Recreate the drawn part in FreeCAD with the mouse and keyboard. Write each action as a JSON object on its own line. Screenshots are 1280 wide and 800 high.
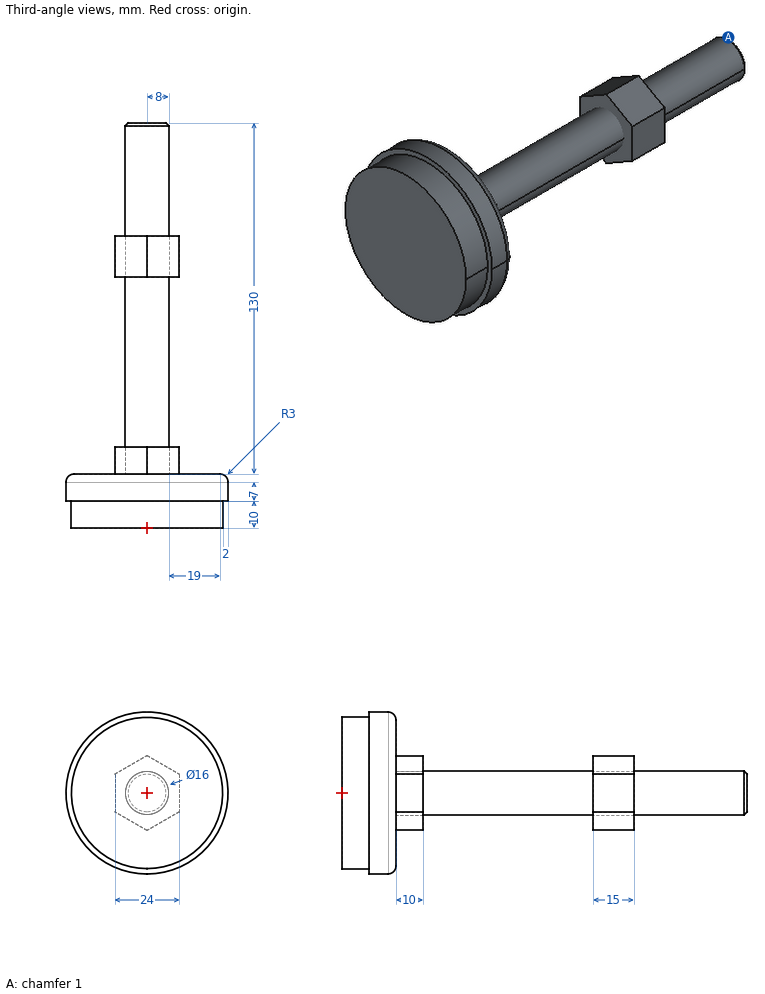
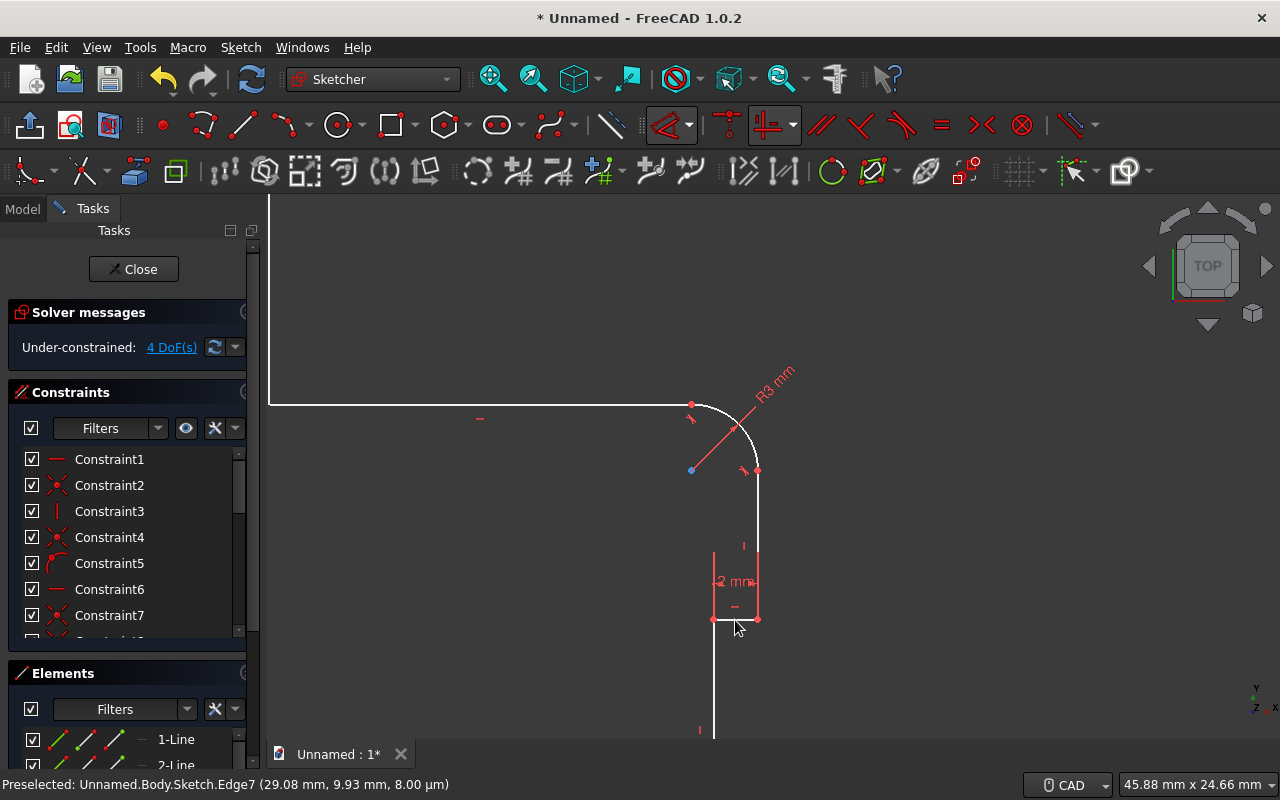
{"action": "scroll", "coordinate": [739, 627], "scroll_direction": "down", "scroll_amount": 11}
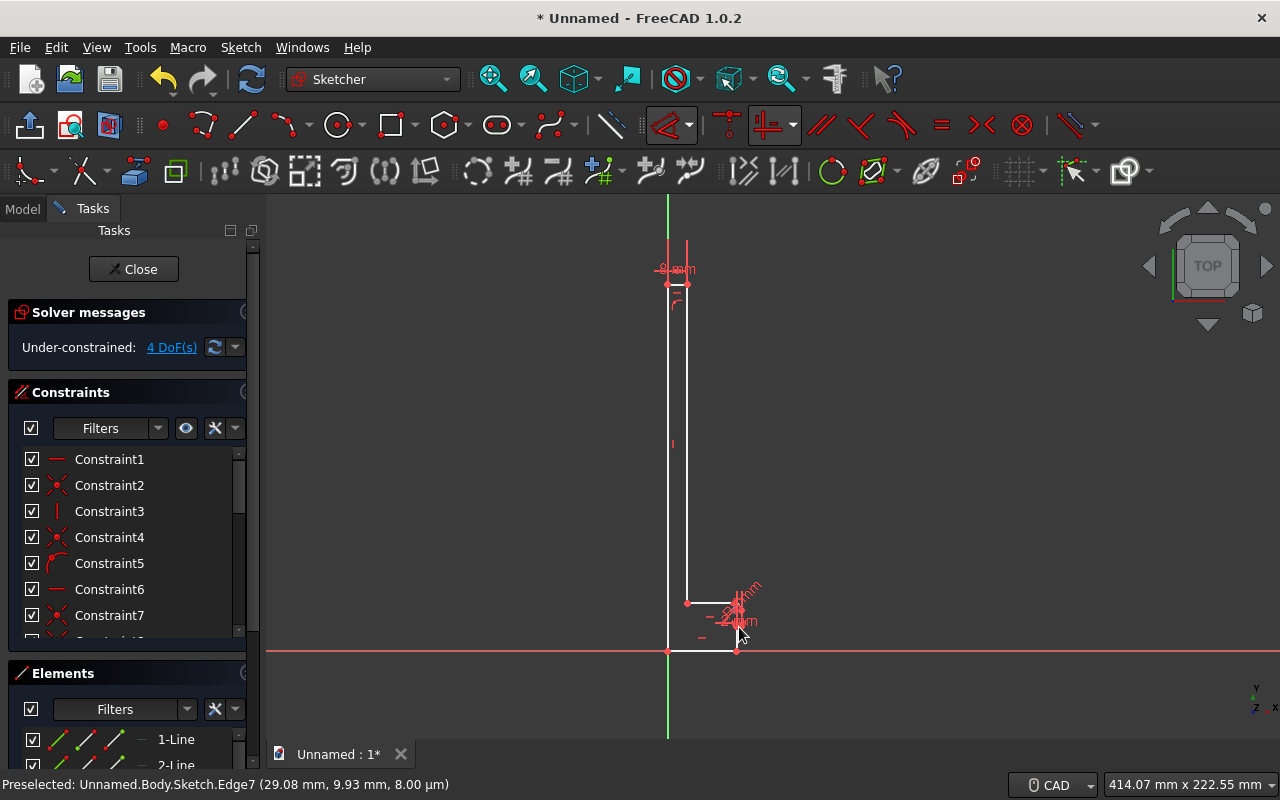
{"action": "scroll", "coordinate": [742, 622], "scroll_direction": "up", "scroll_amount": 6}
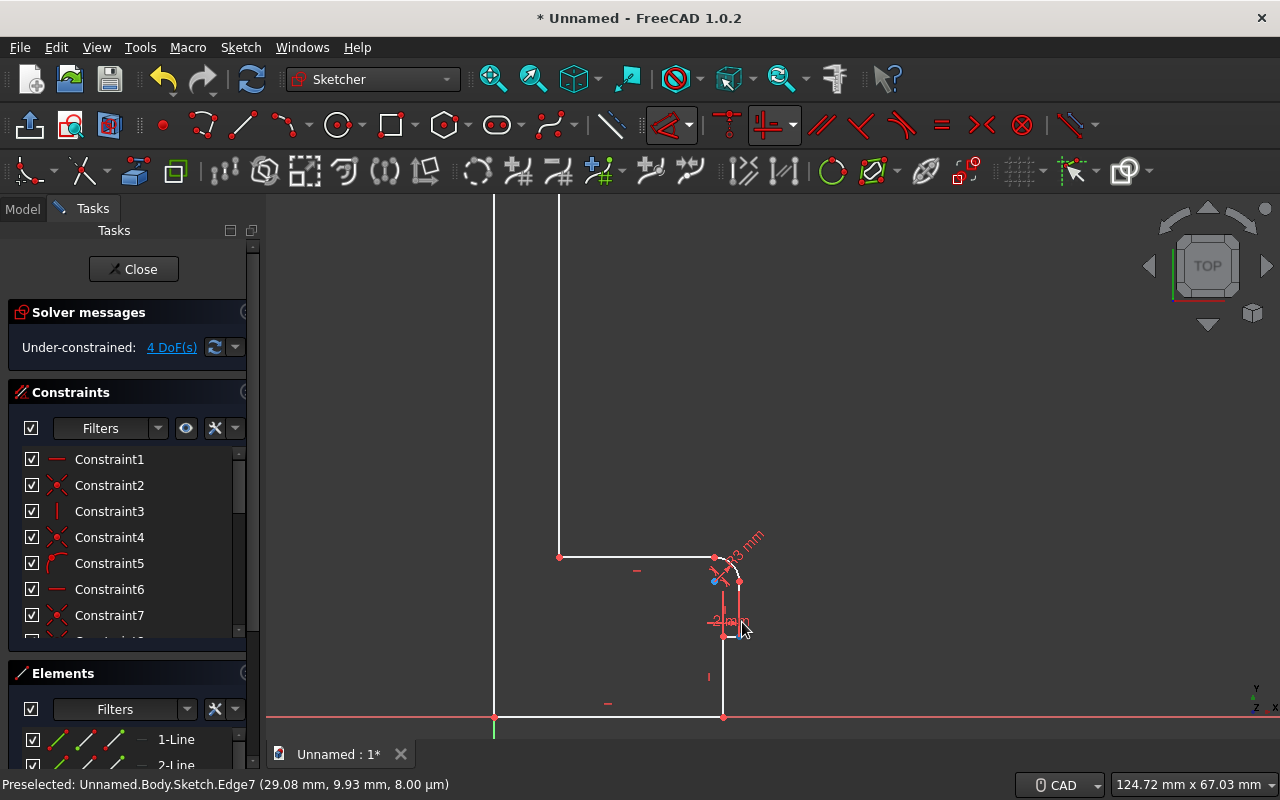
{"action": "left_click", "coordinate": [739, 598]}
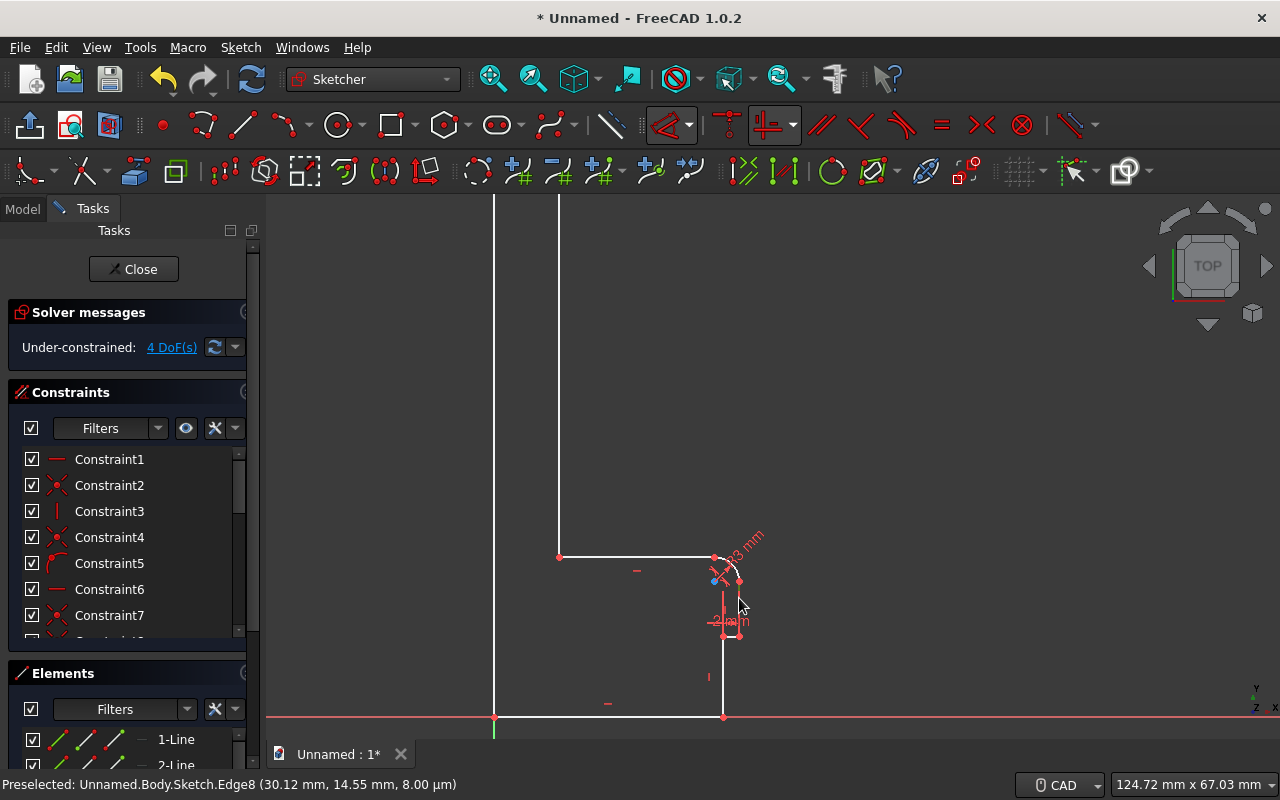
{"action": "left_click", "coordinate": [692, 126]}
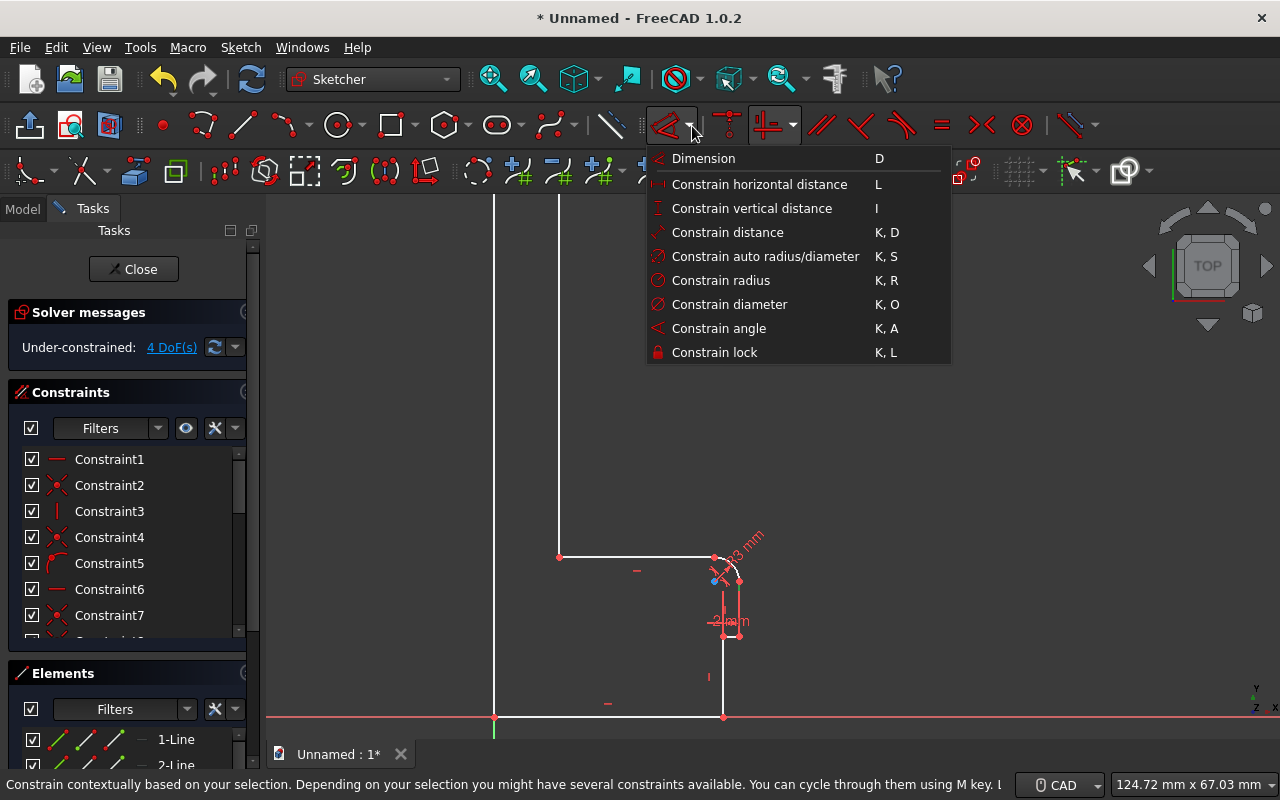
{"action": "left_click", "coordinate": [799, 208]}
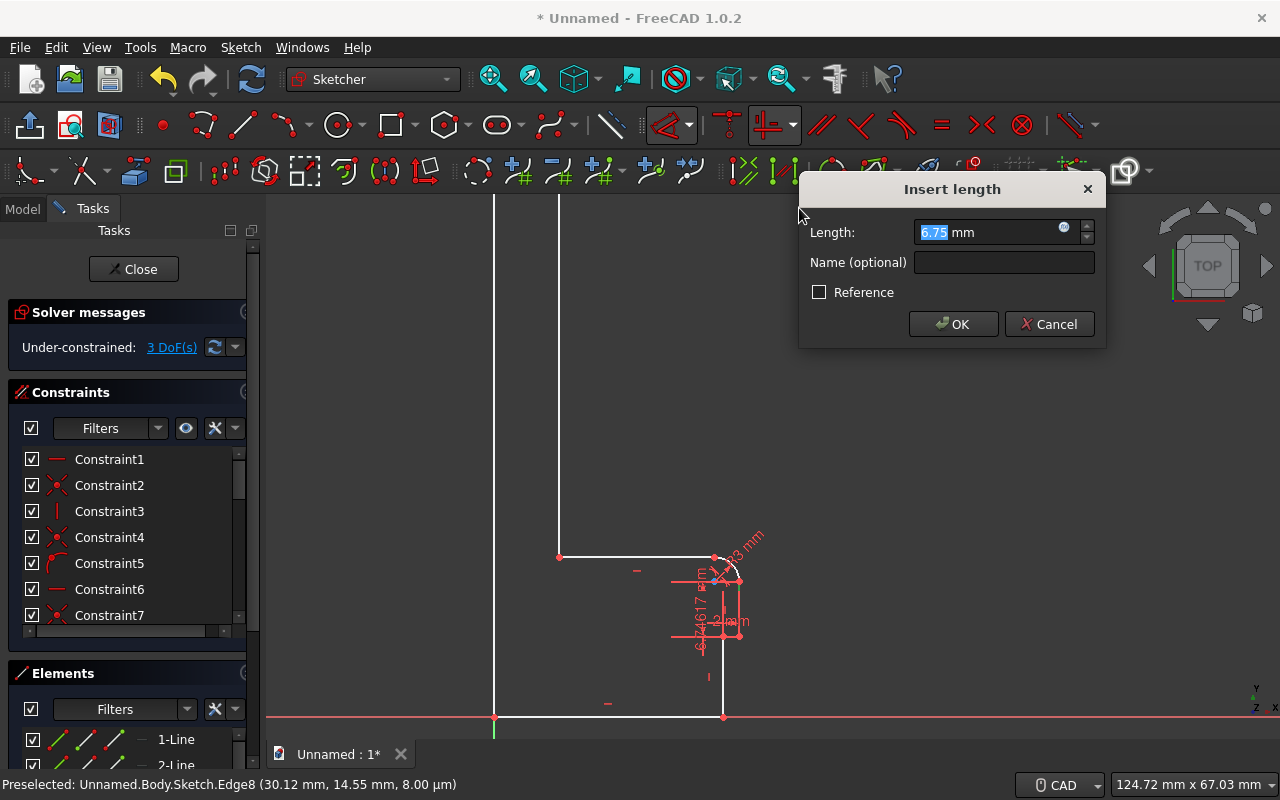
{"action": "type", "text": "7"}
{"action": "key", "text": "Return"}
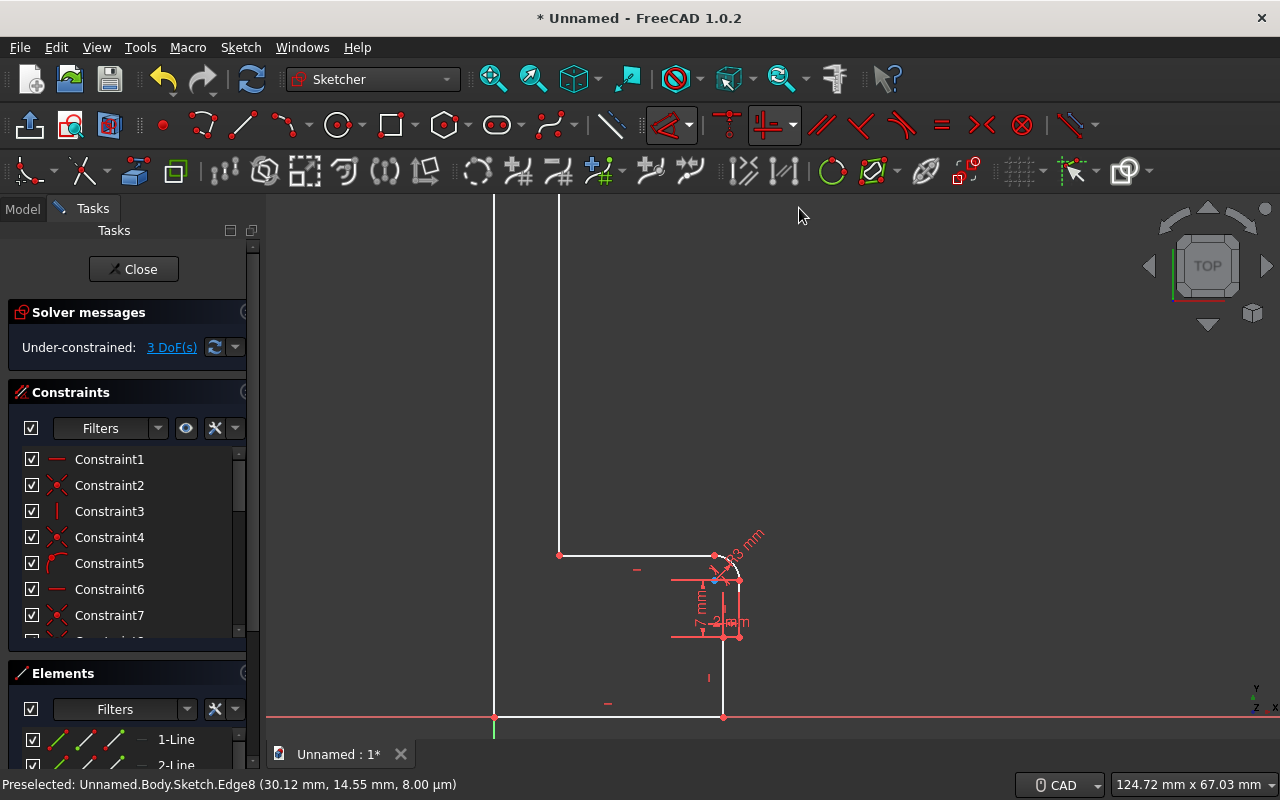
{"action": "scroll", "coordinate": [742, 621], "scroll_direction": "down", "scroll_amount": 6}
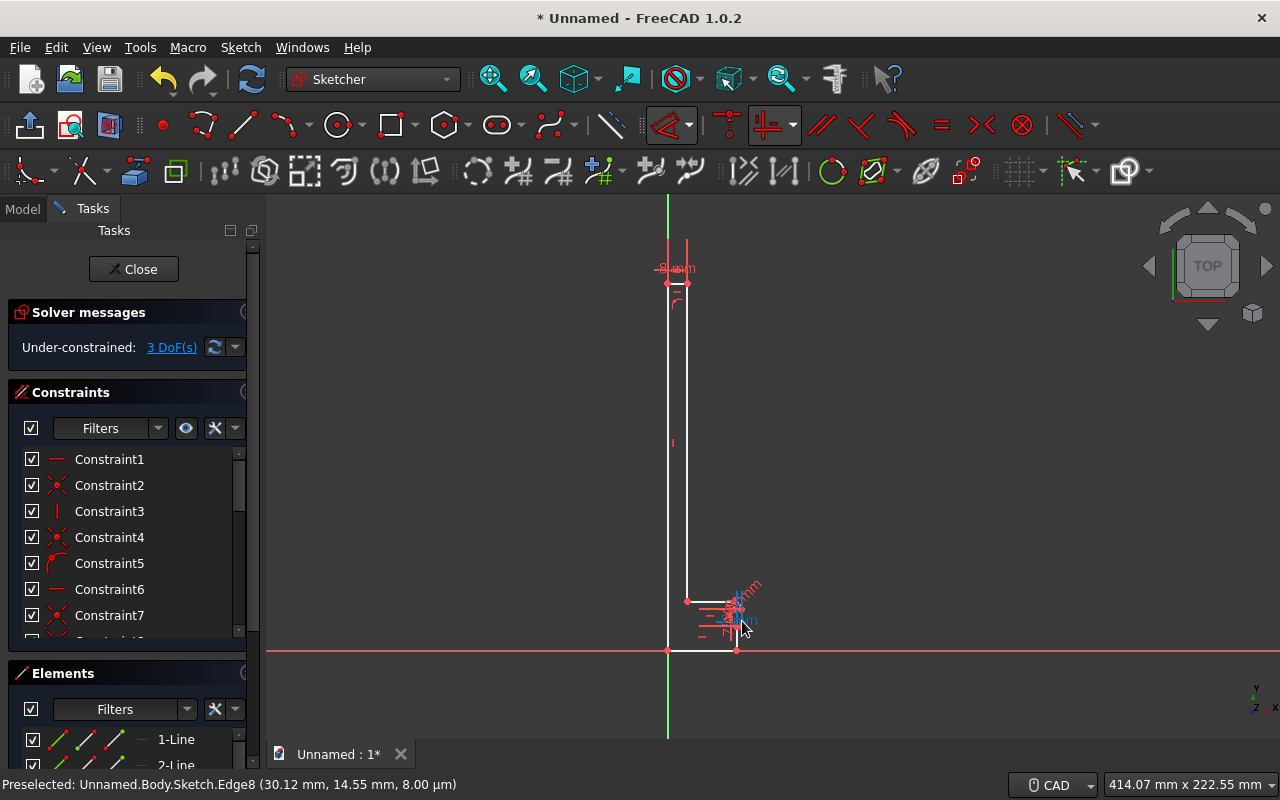
{"action": "left_click", "coordinate": [720, 602]}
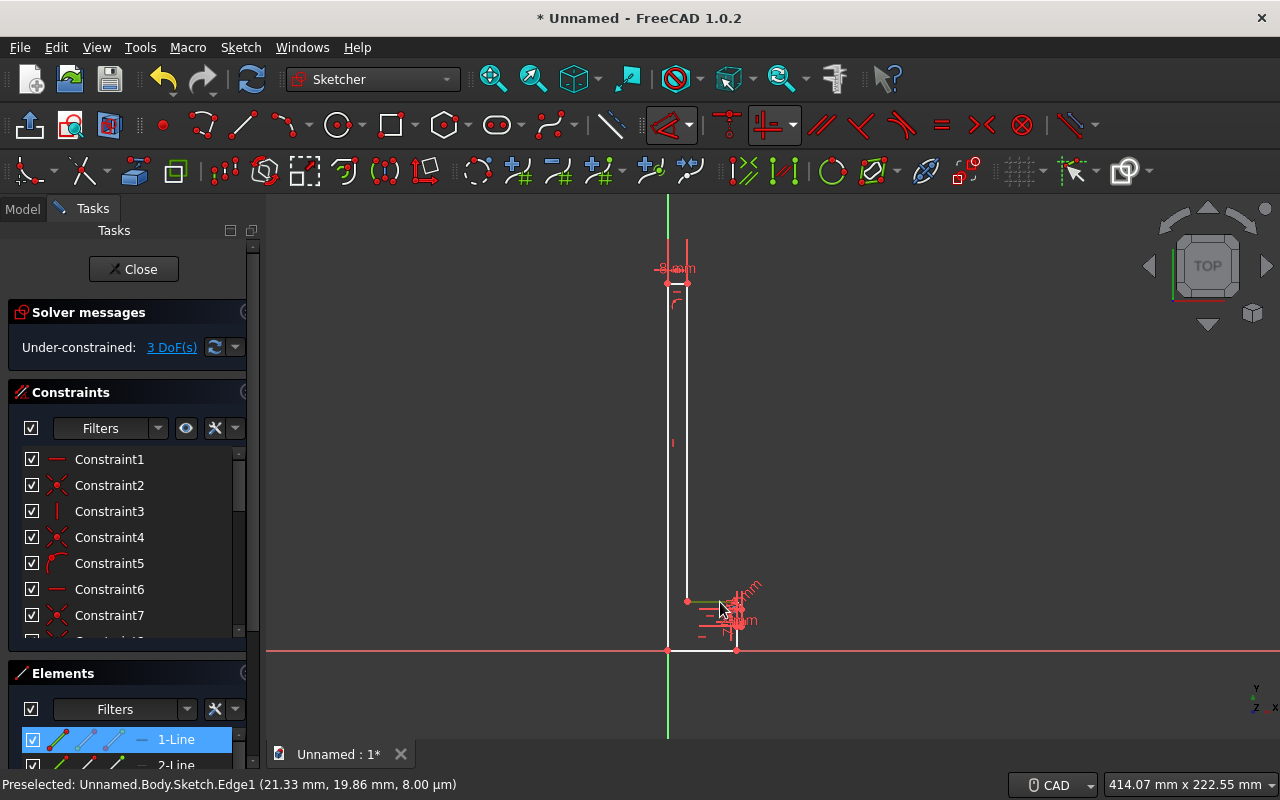
{"action": "left_click", "coordinate": [692, 126]}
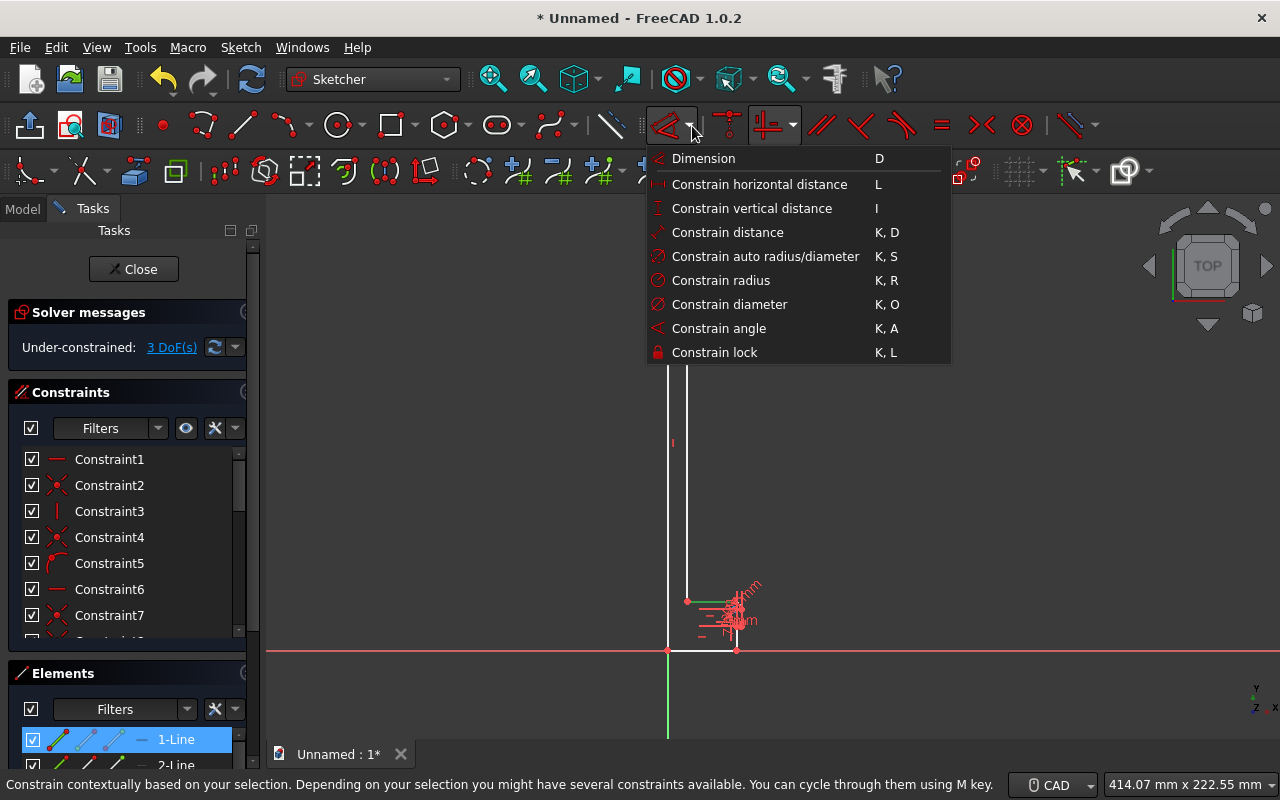
{"action": "left_click", "coordinate": [799, 184]}